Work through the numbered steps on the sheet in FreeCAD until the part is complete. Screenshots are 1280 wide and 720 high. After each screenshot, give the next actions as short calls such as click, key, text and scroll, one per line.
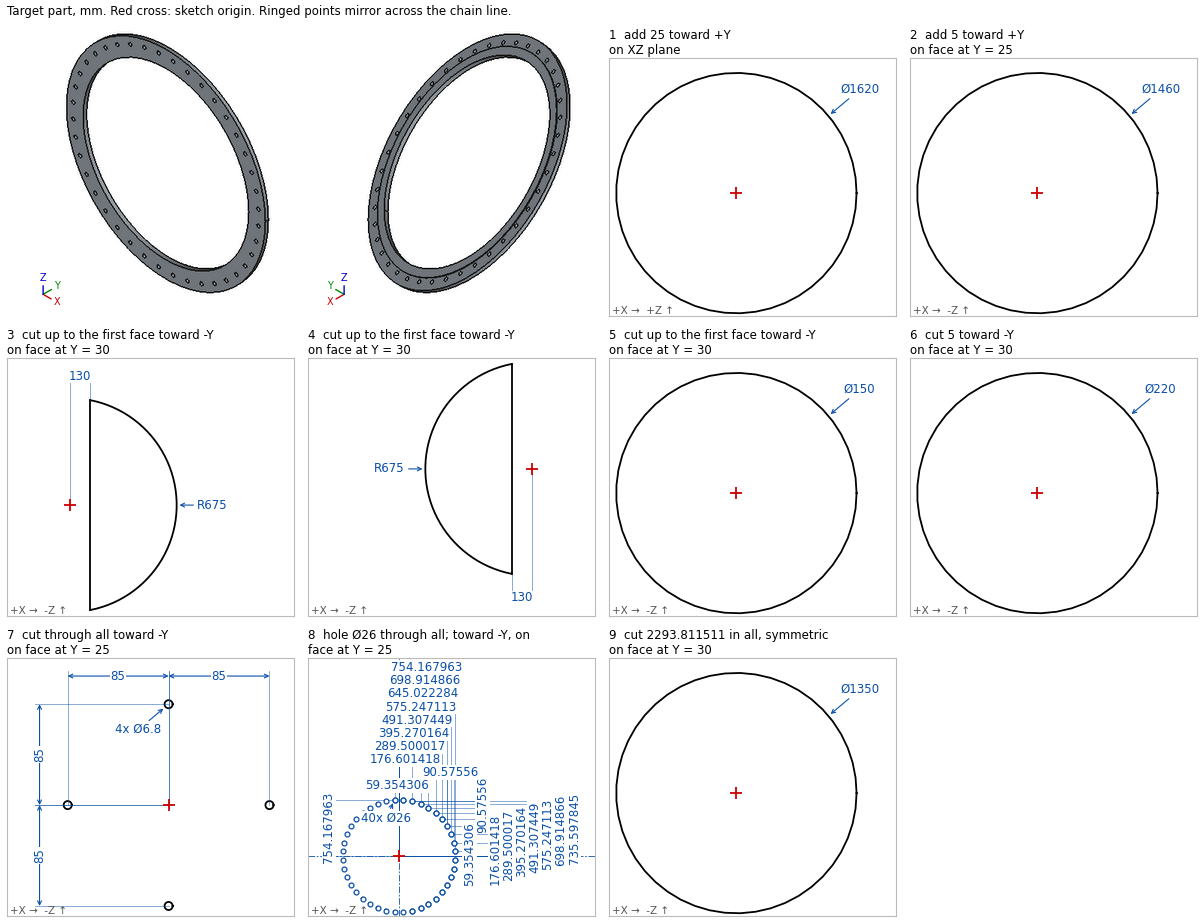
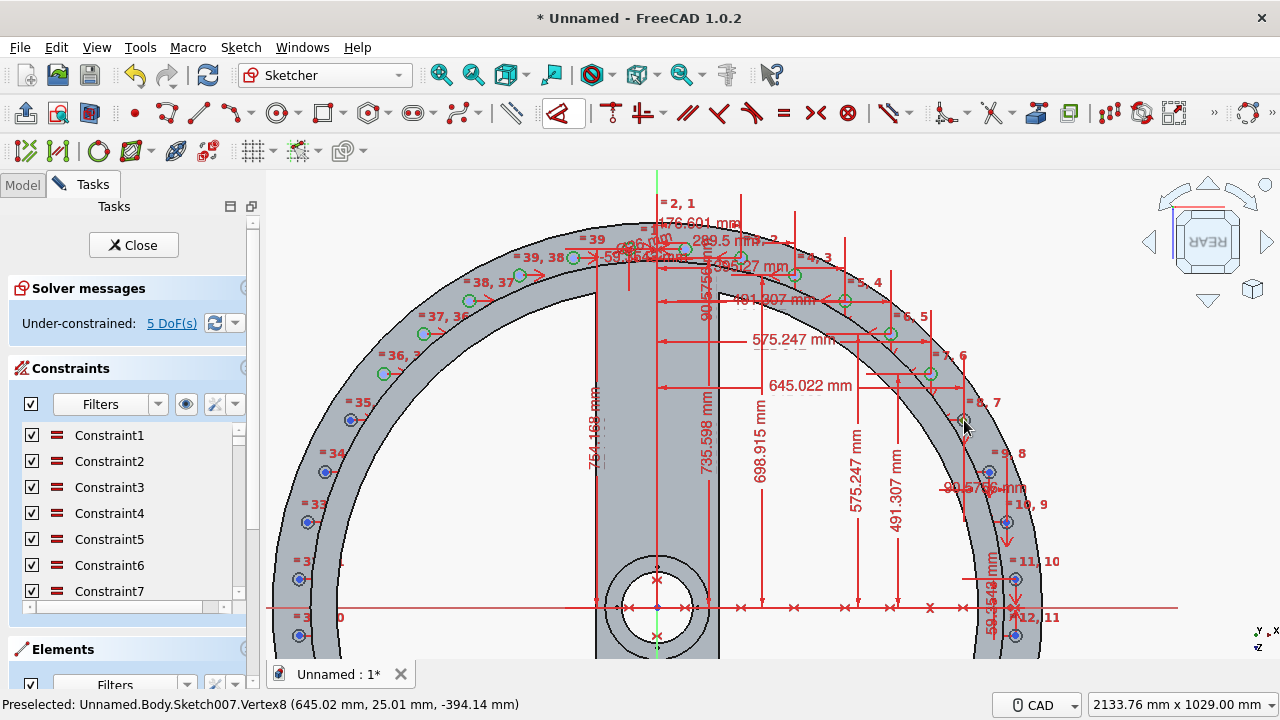
key(i)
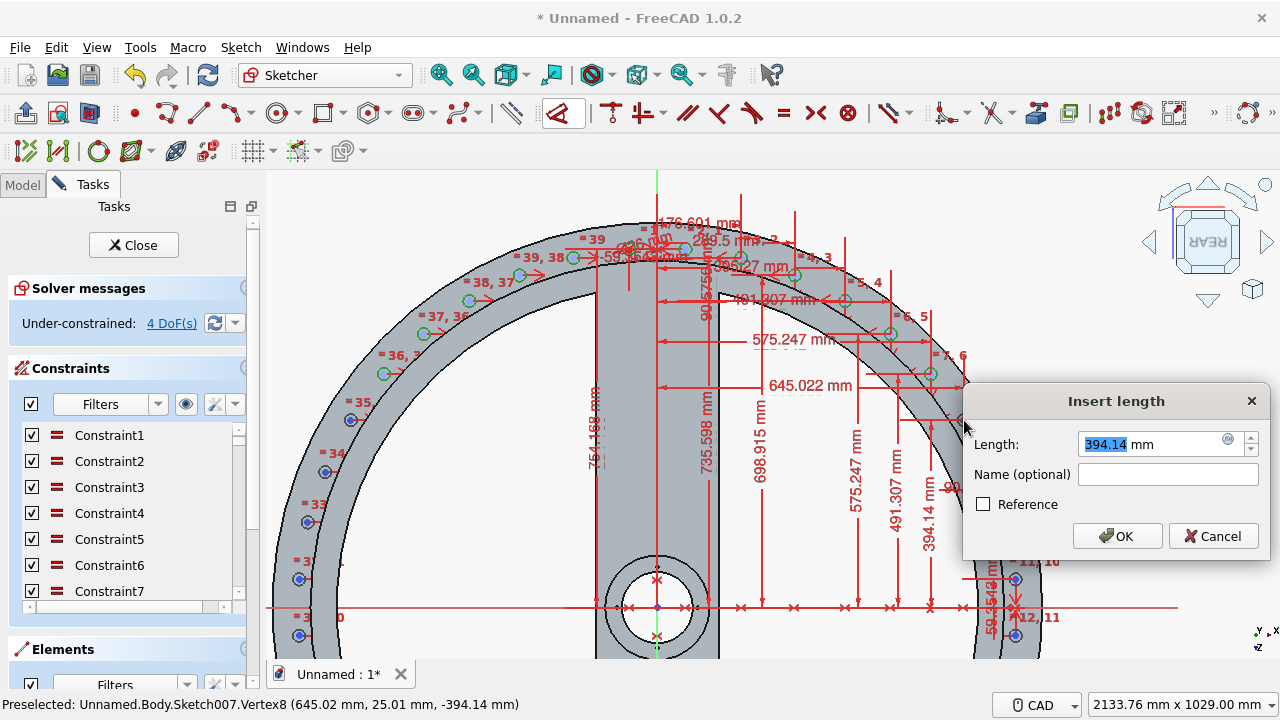
text(395.270164)
key(Return)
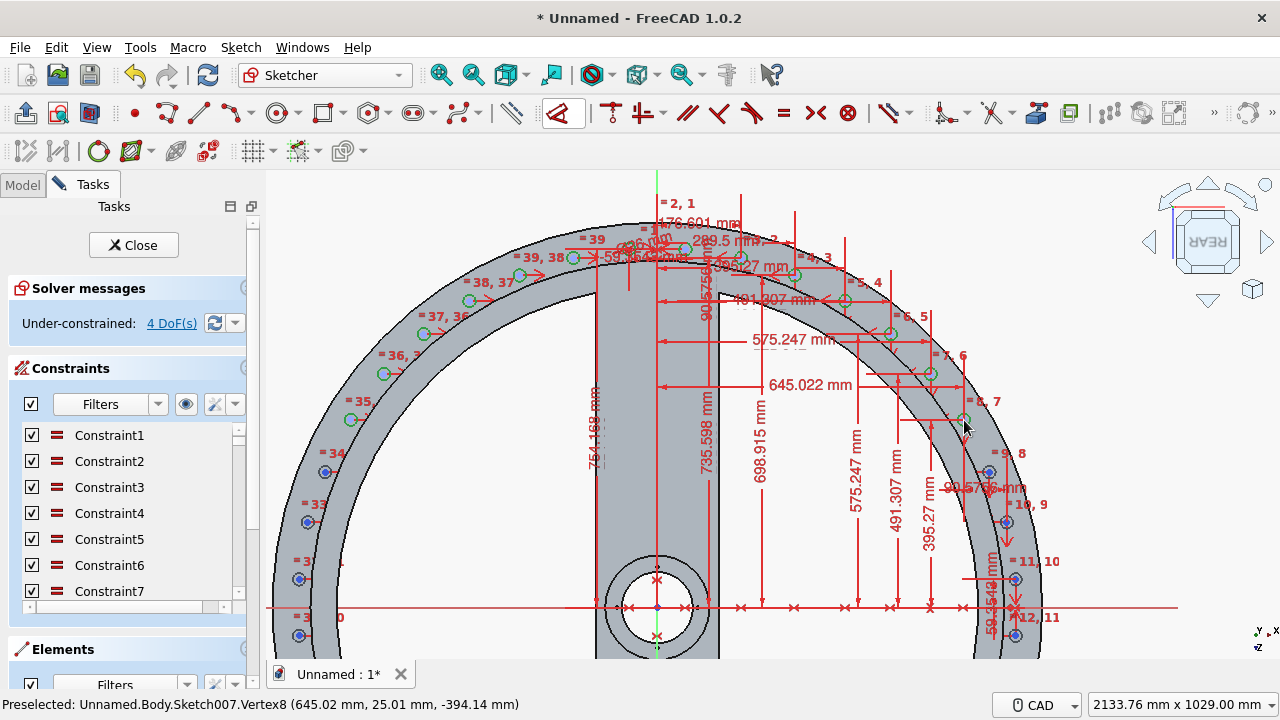
click(989, 472)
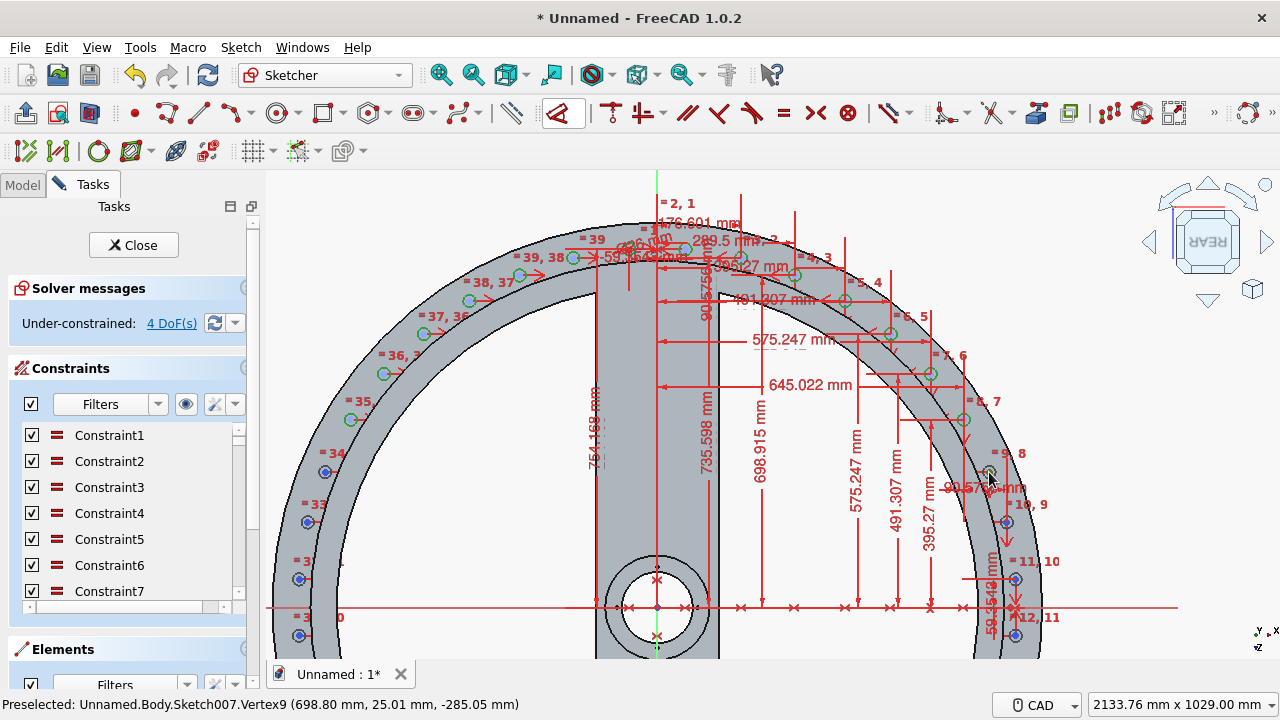
key(l)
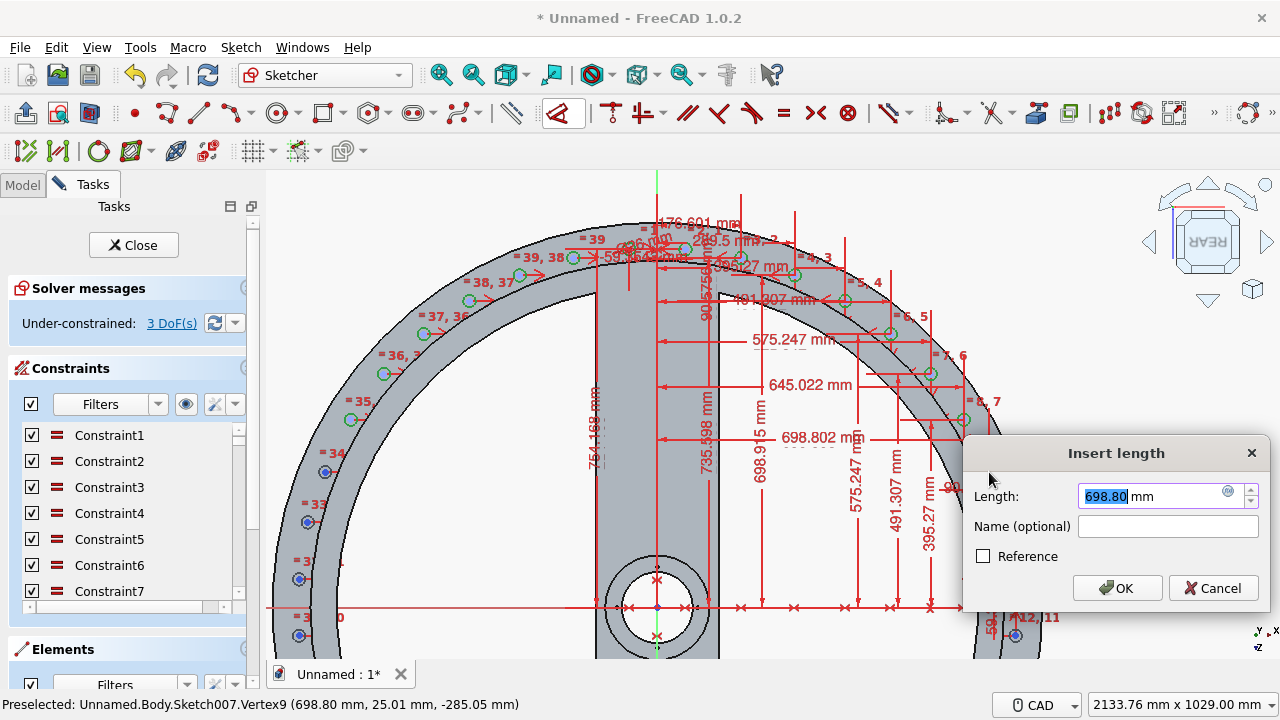
text(698.914866)
key(Return)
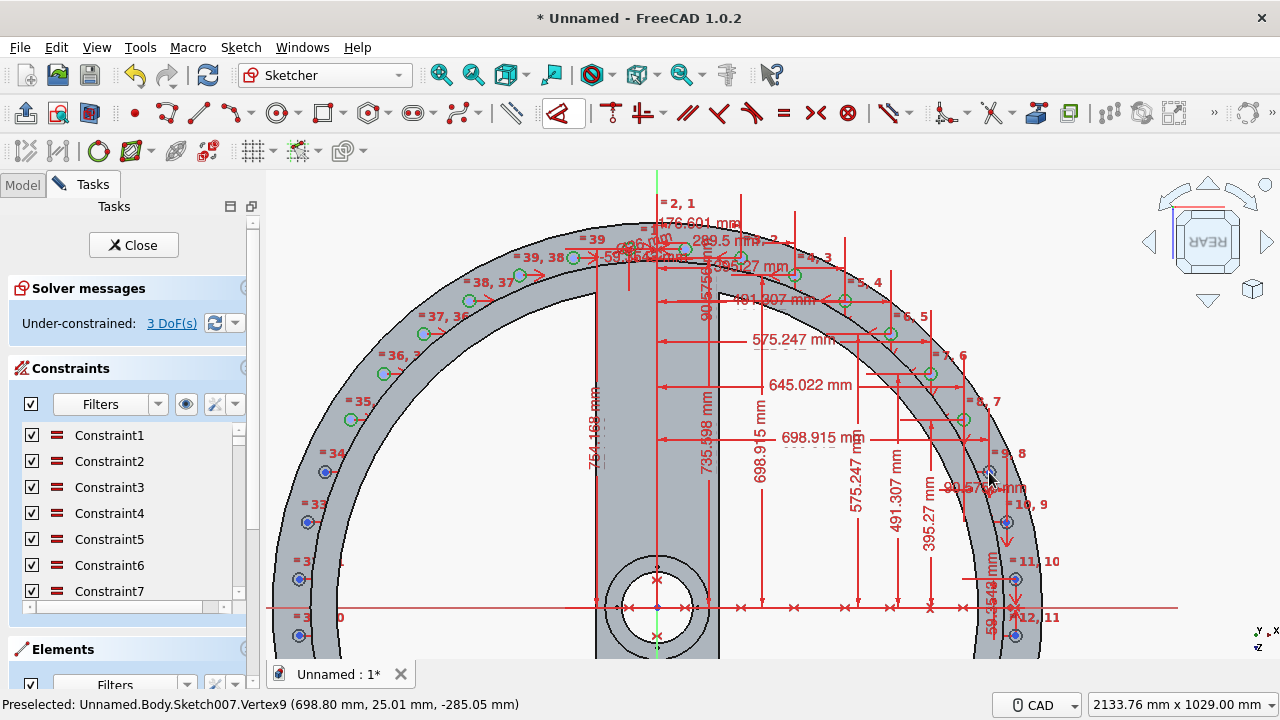
click(989, 472)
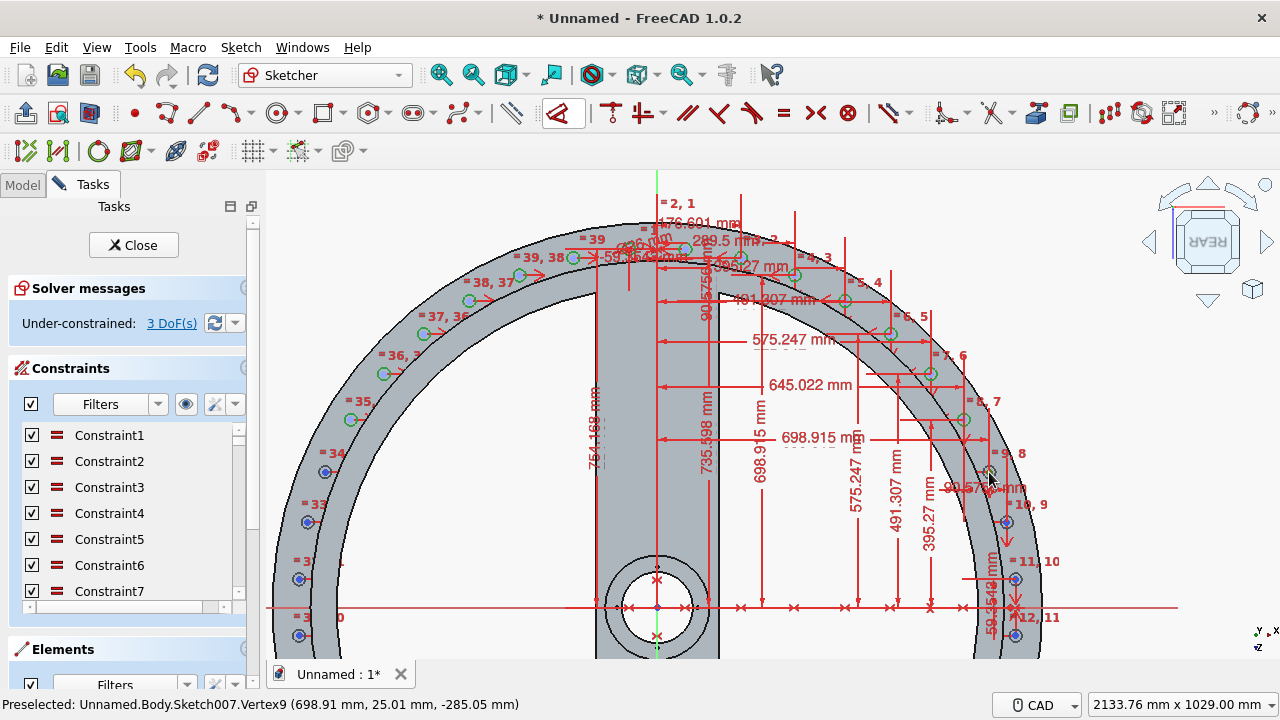
click(580, 114)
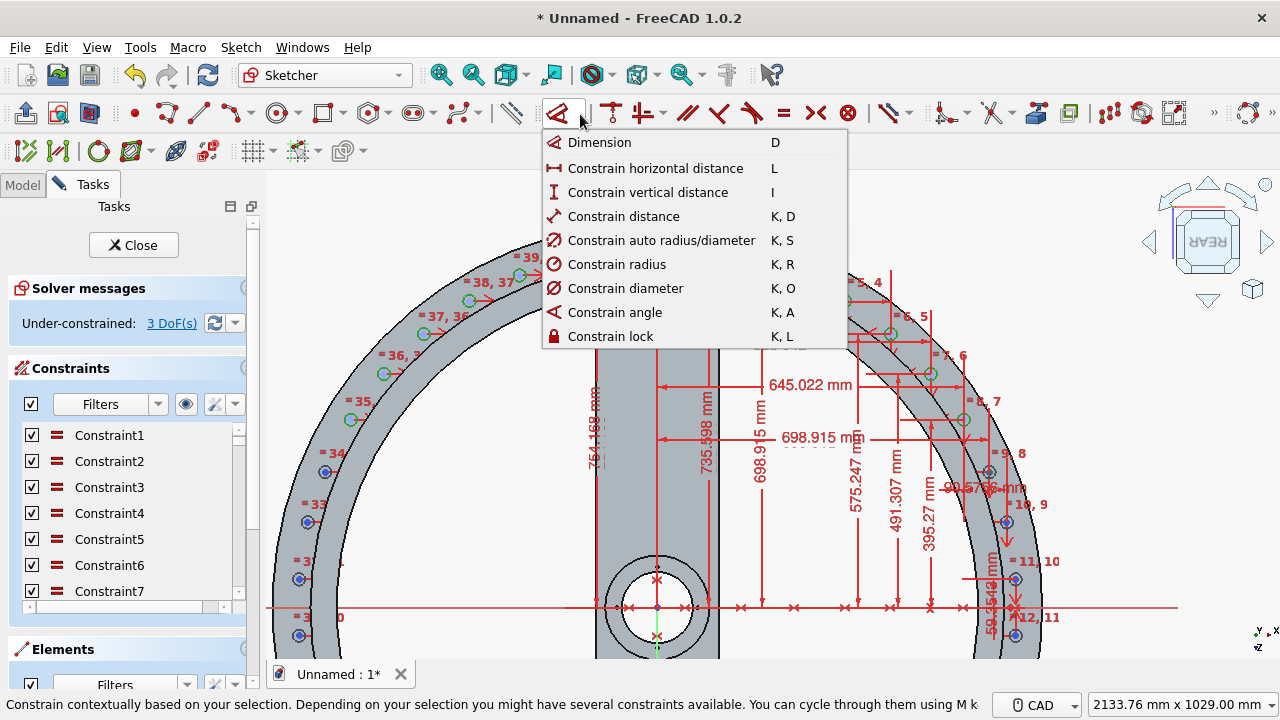
click(695, 192)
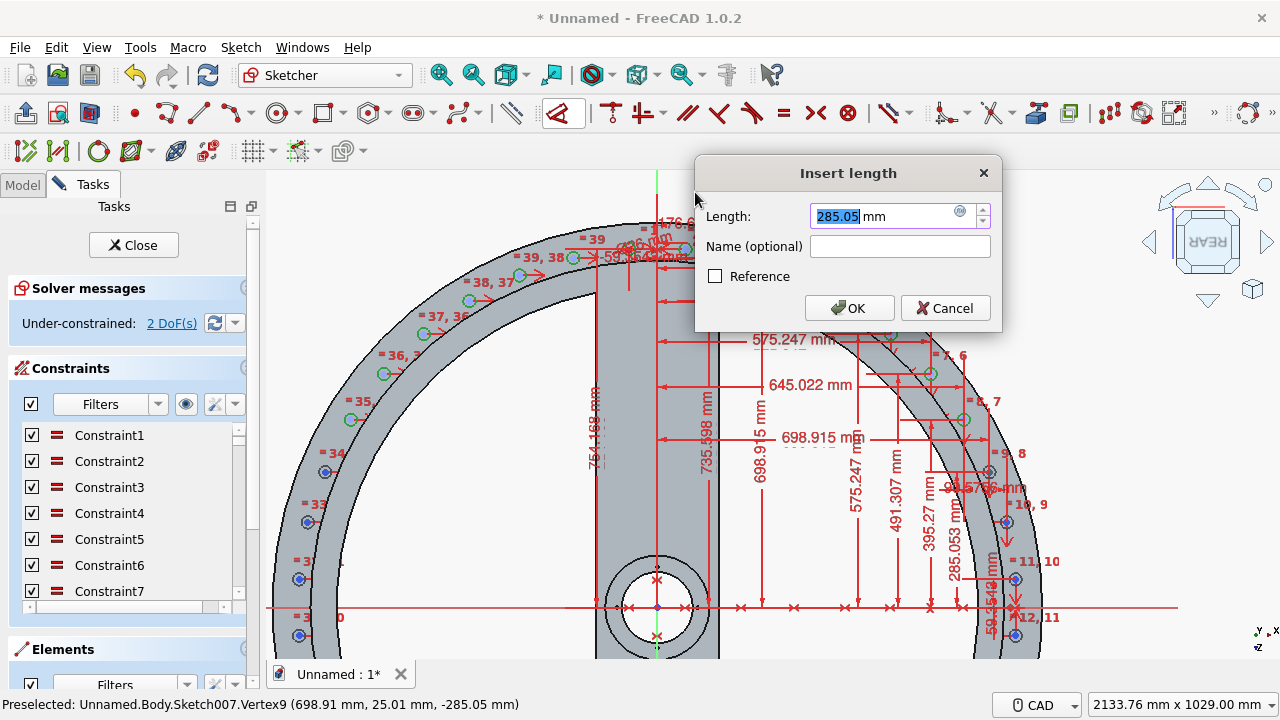
text(289.500017)
key(Return)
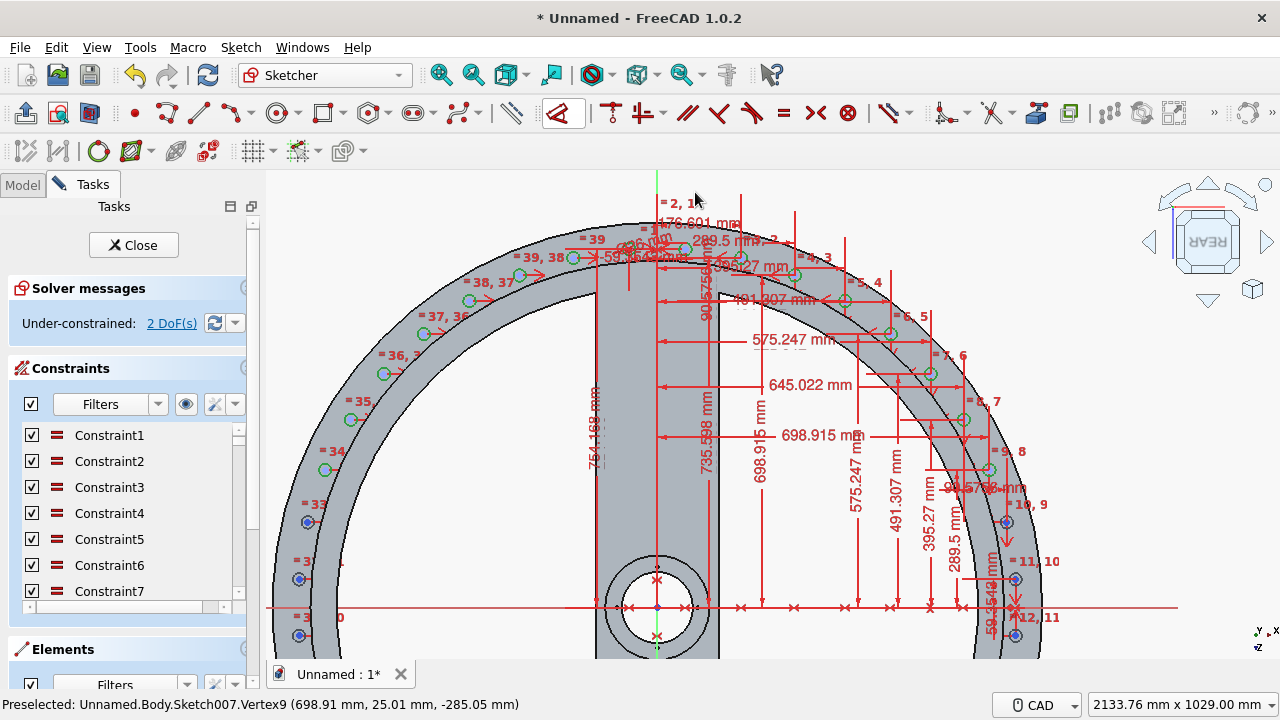
click(1007, 522)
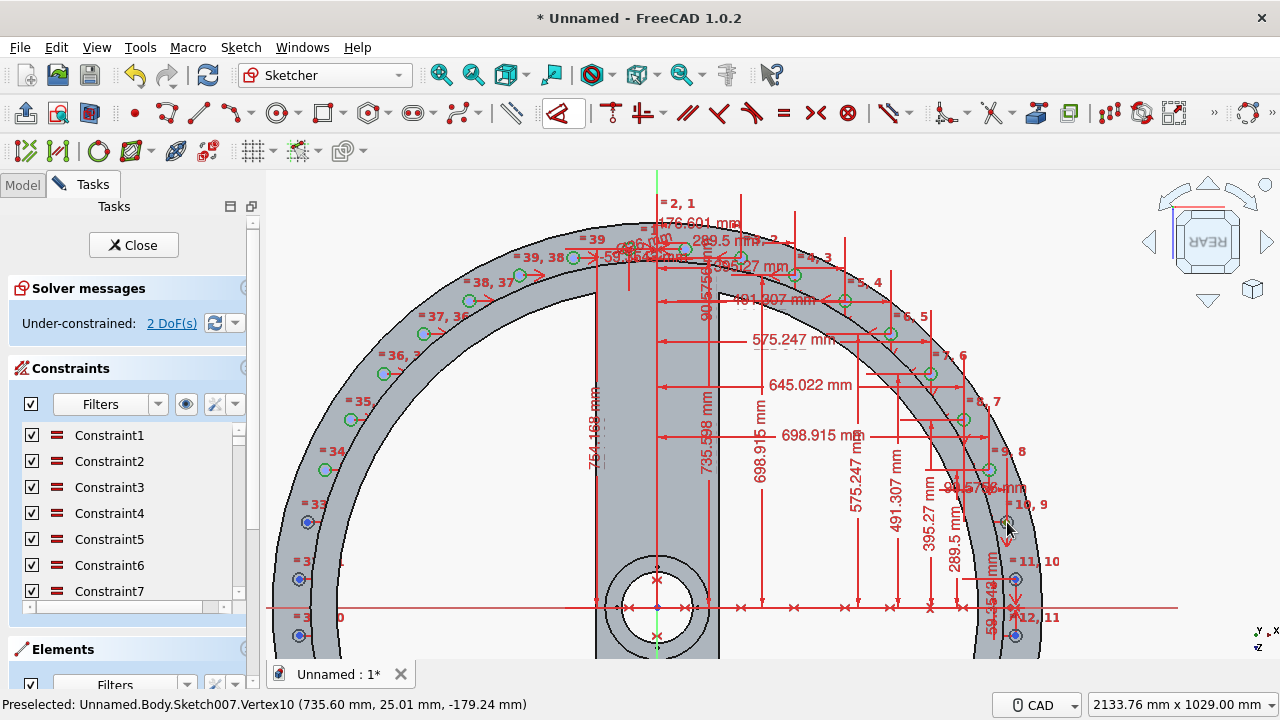
key(i)